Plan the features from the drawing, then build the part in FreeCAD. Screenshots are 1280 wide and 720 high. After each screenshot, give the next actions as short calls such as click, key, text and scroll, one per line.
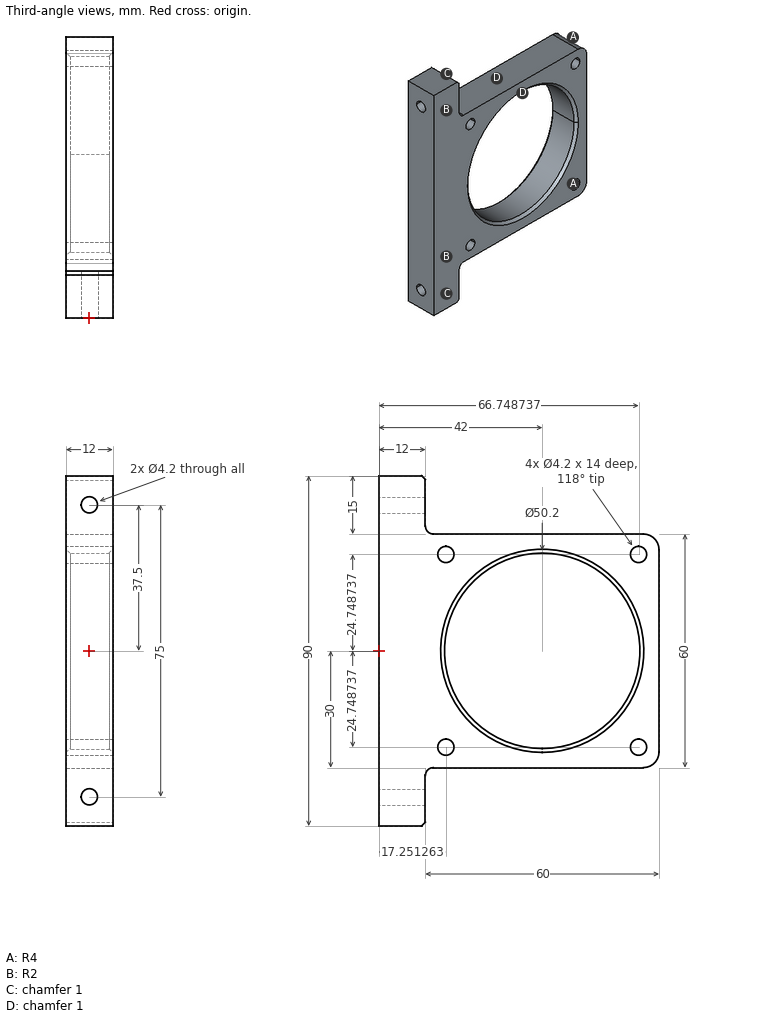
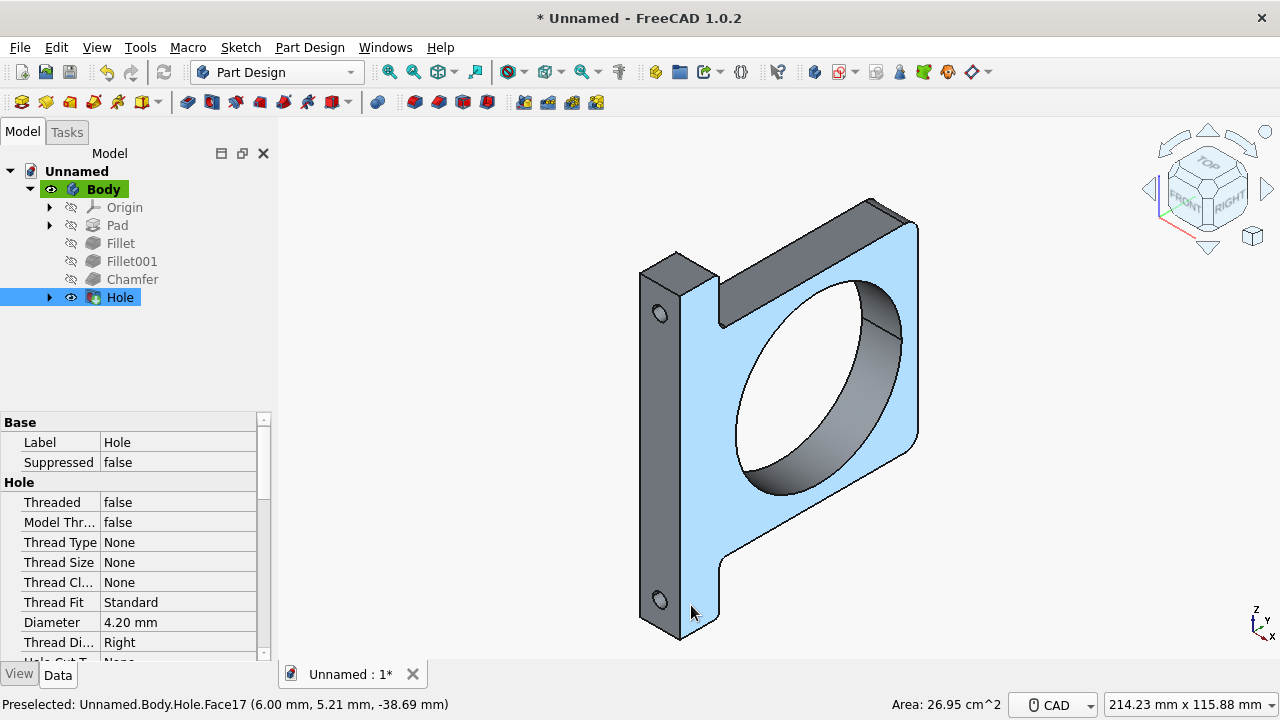
click(840, 72)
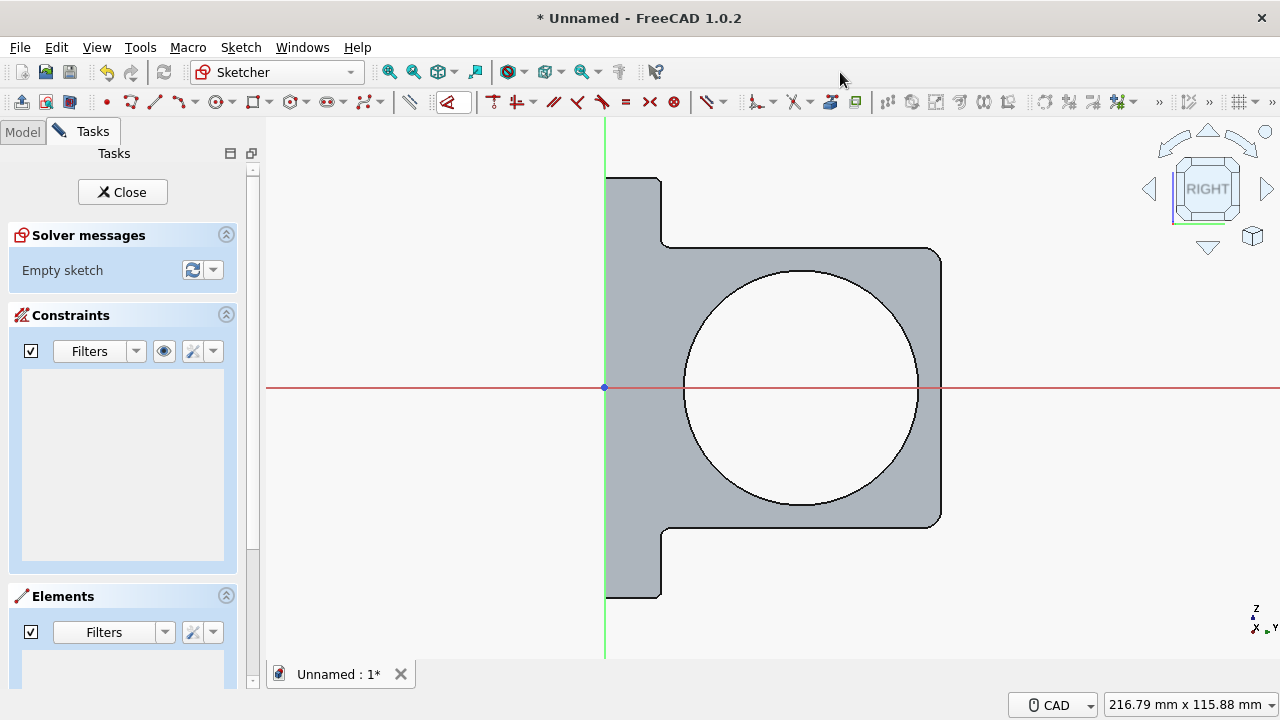
scroll(890, 388, up, 2)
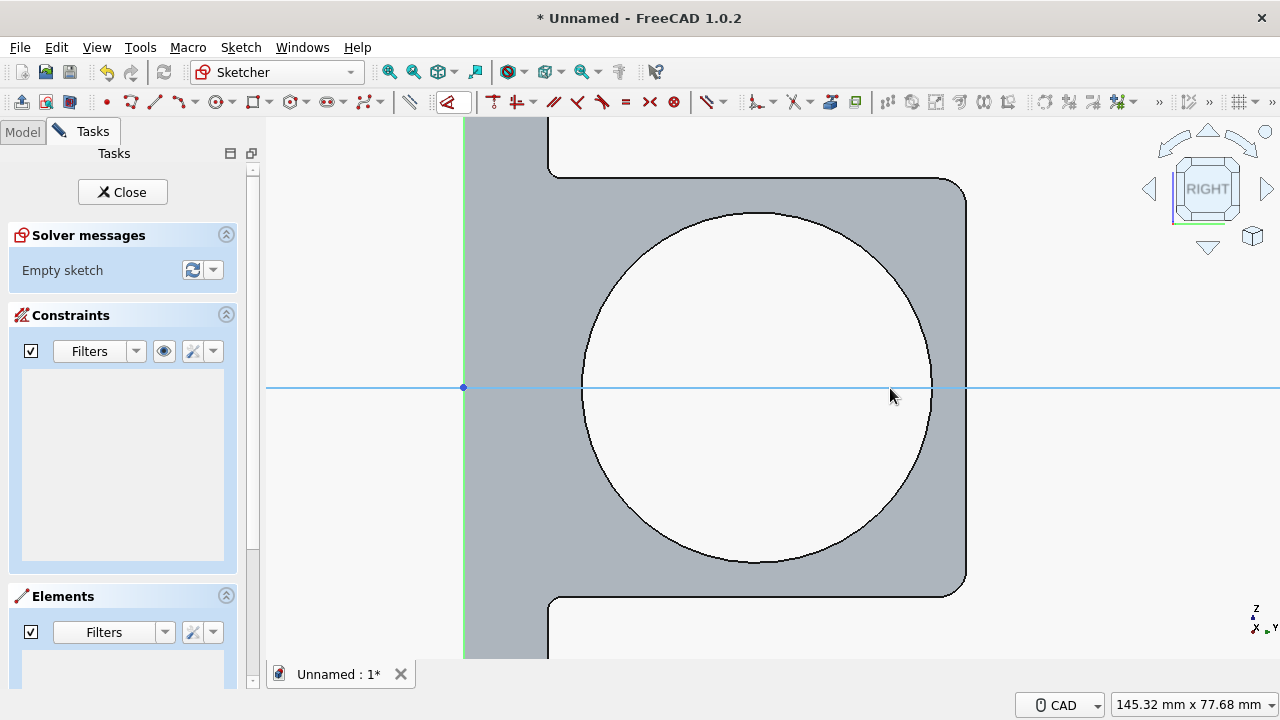
click(216, 102)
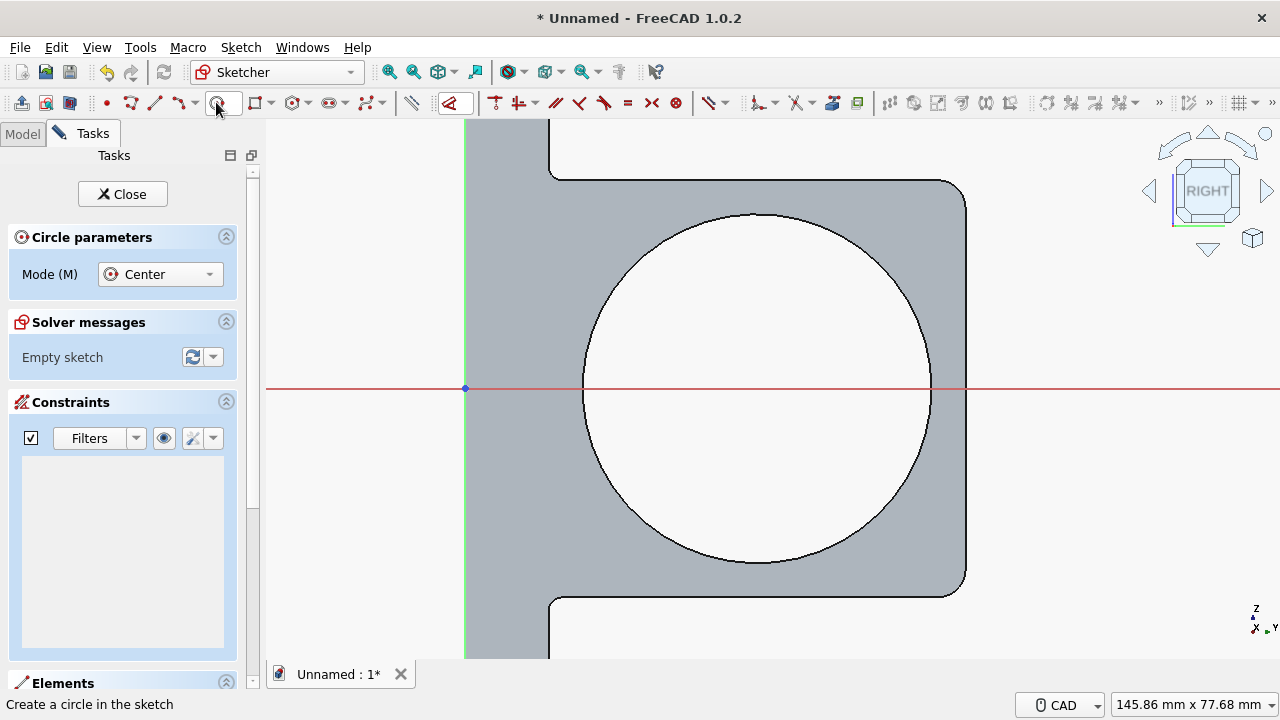
scroll(929, 217, up, 3)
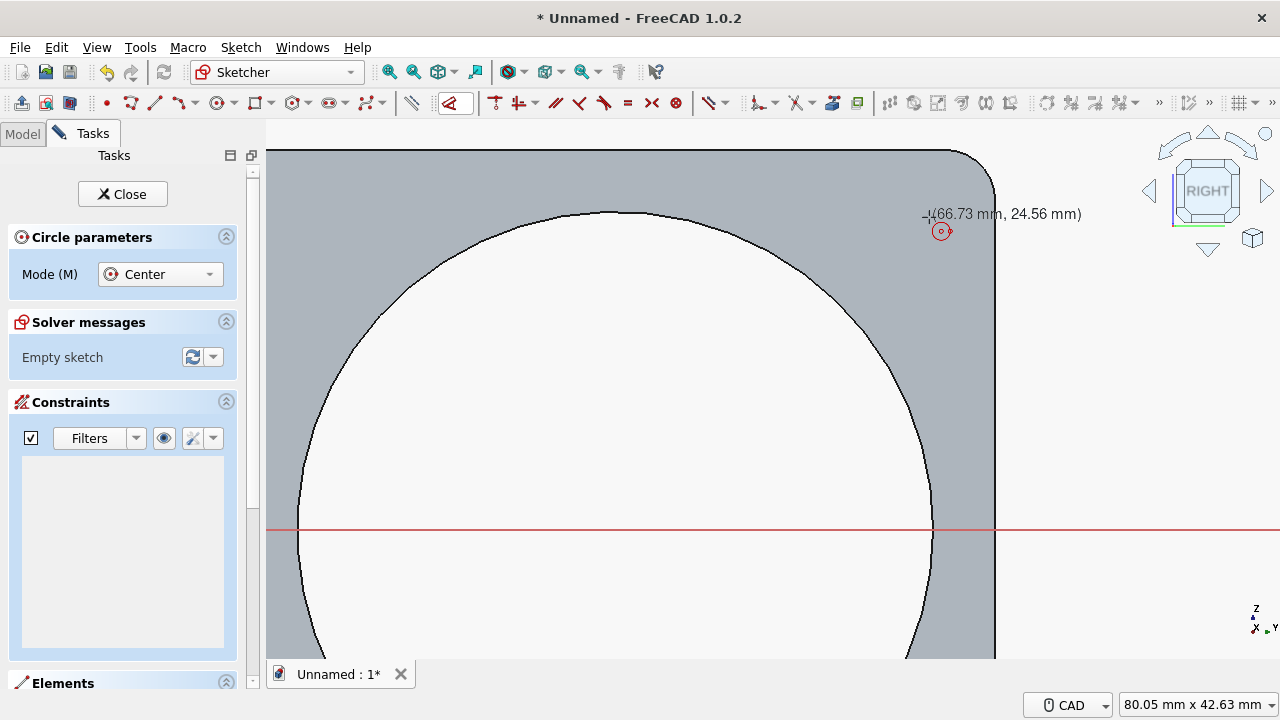
click(929, 216)
move(948, 197)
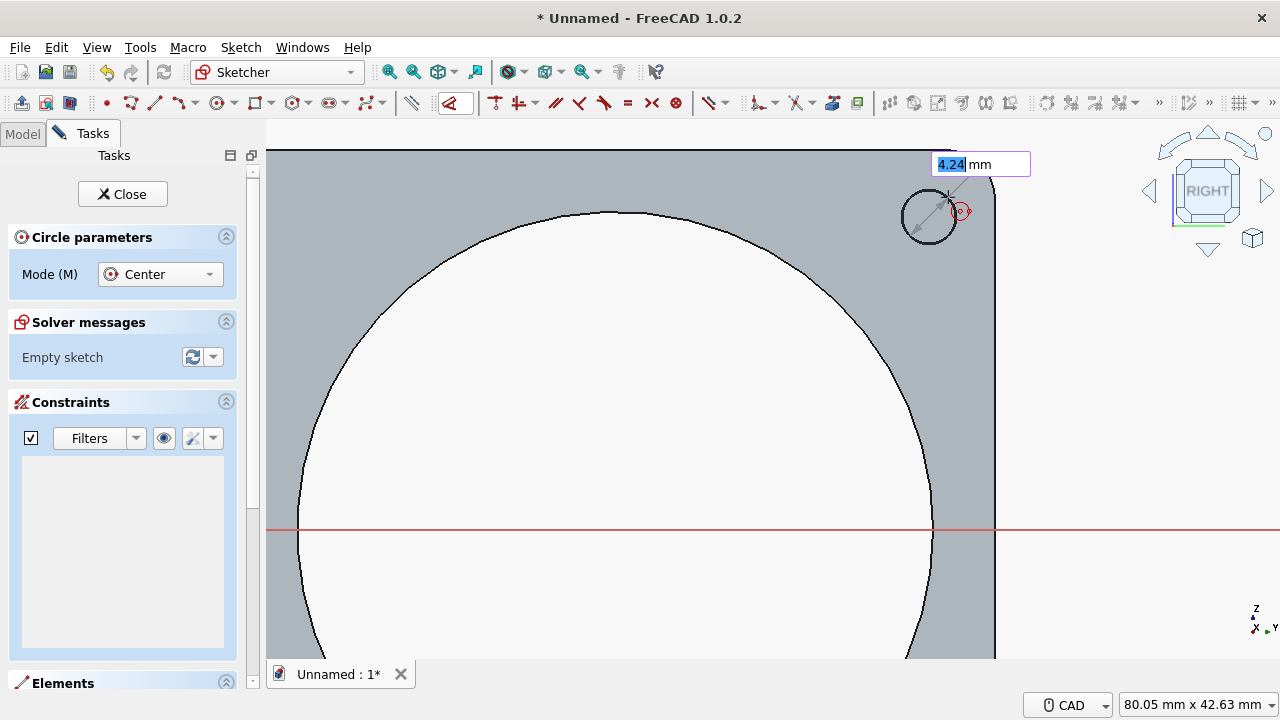
text(4.2)
key(Return)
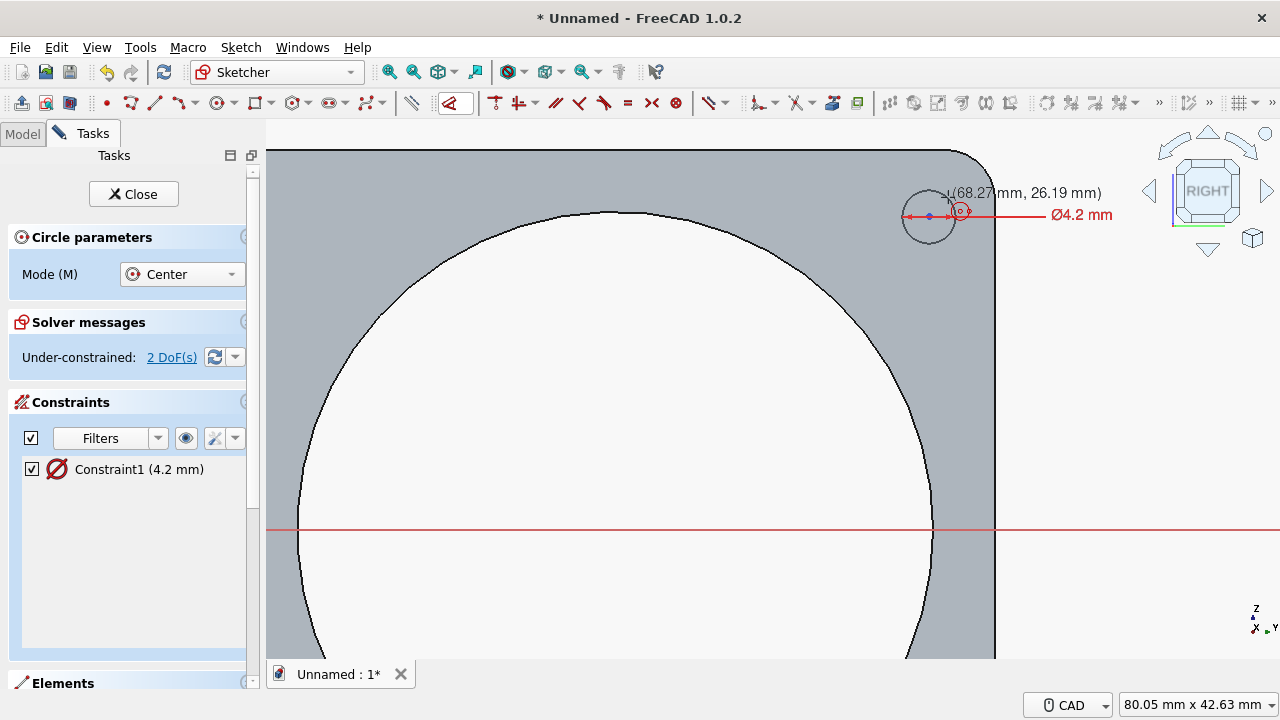
scroll(930, 218, down, 3)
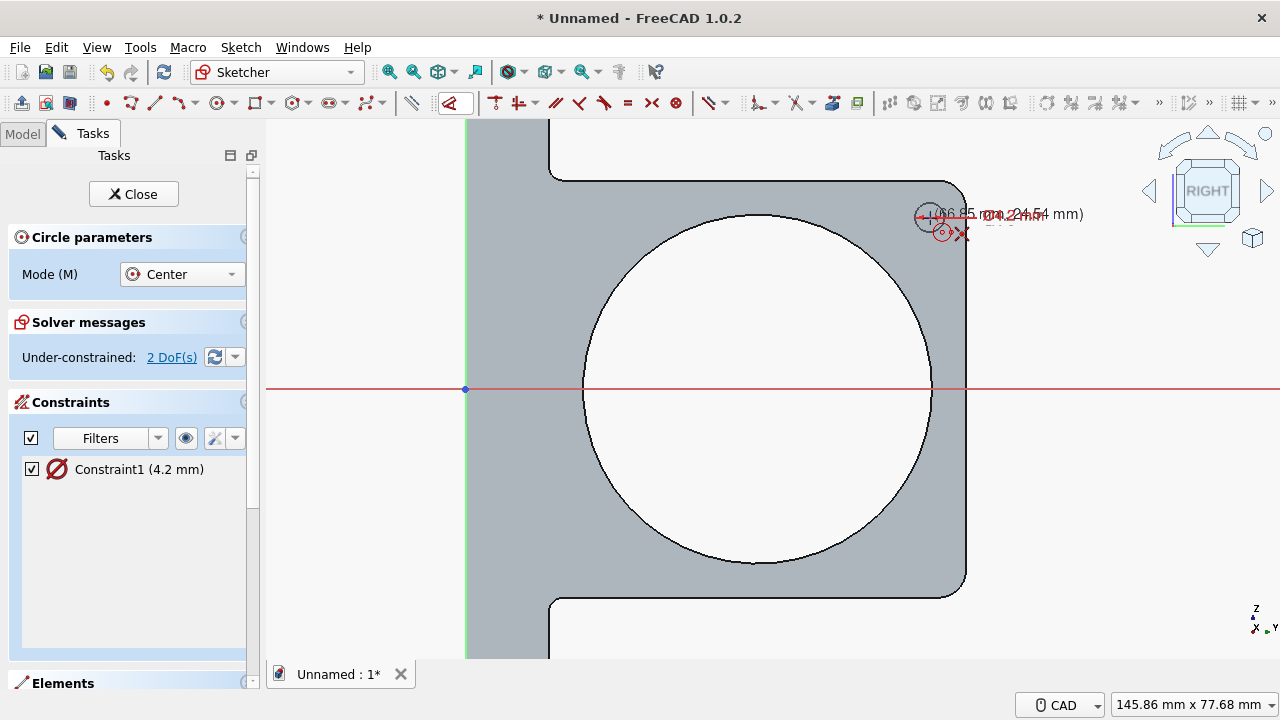
scroll(930, 561, up, 3)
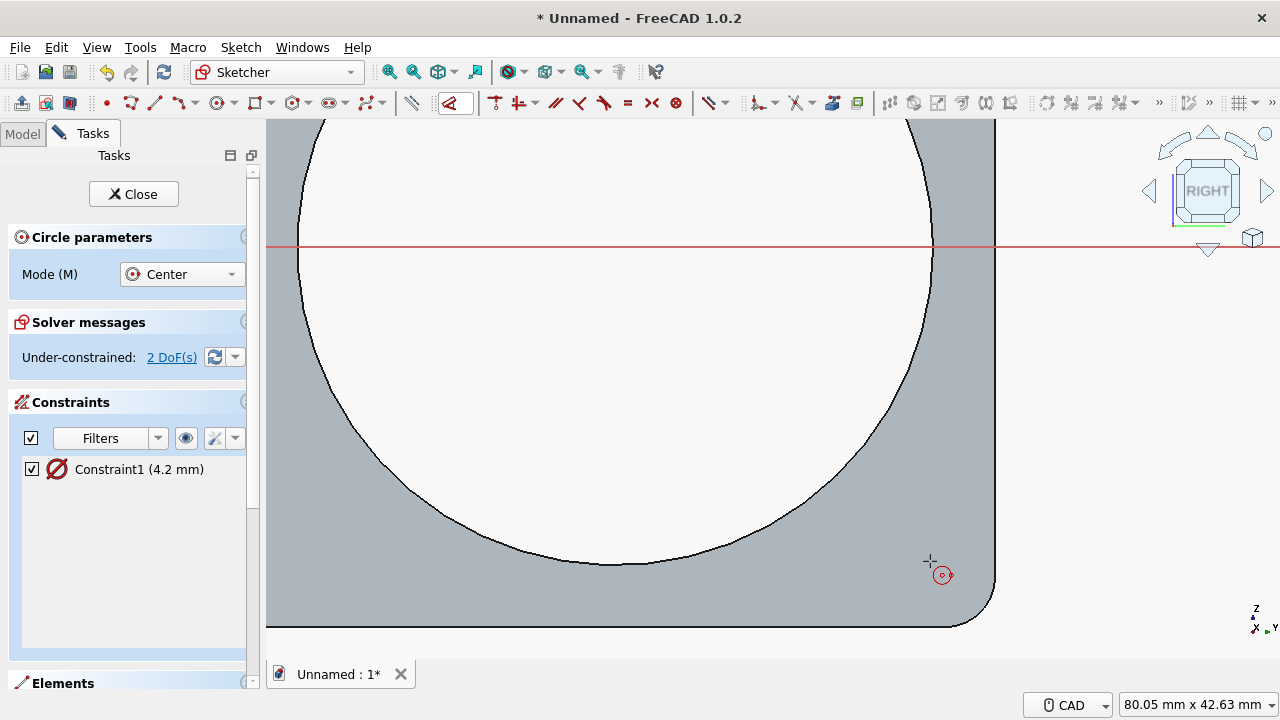
click(929, 561)
move(948, 542)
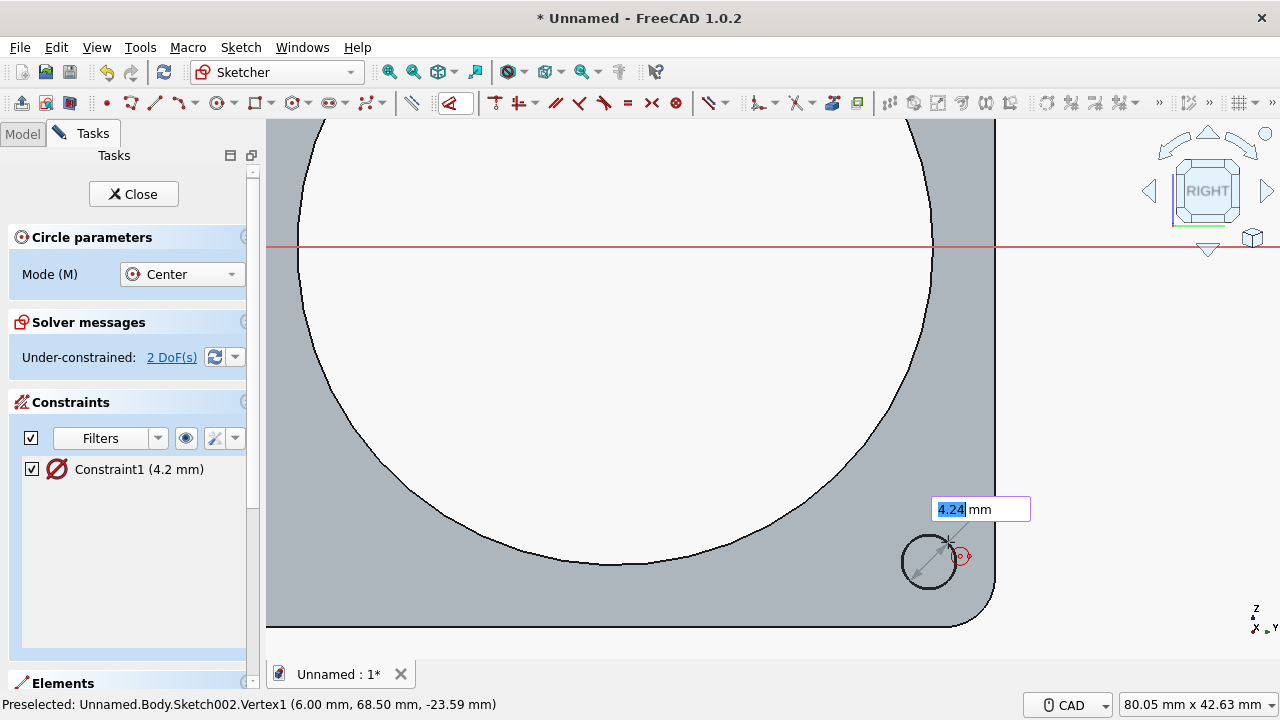
text(4.2)
key(Return)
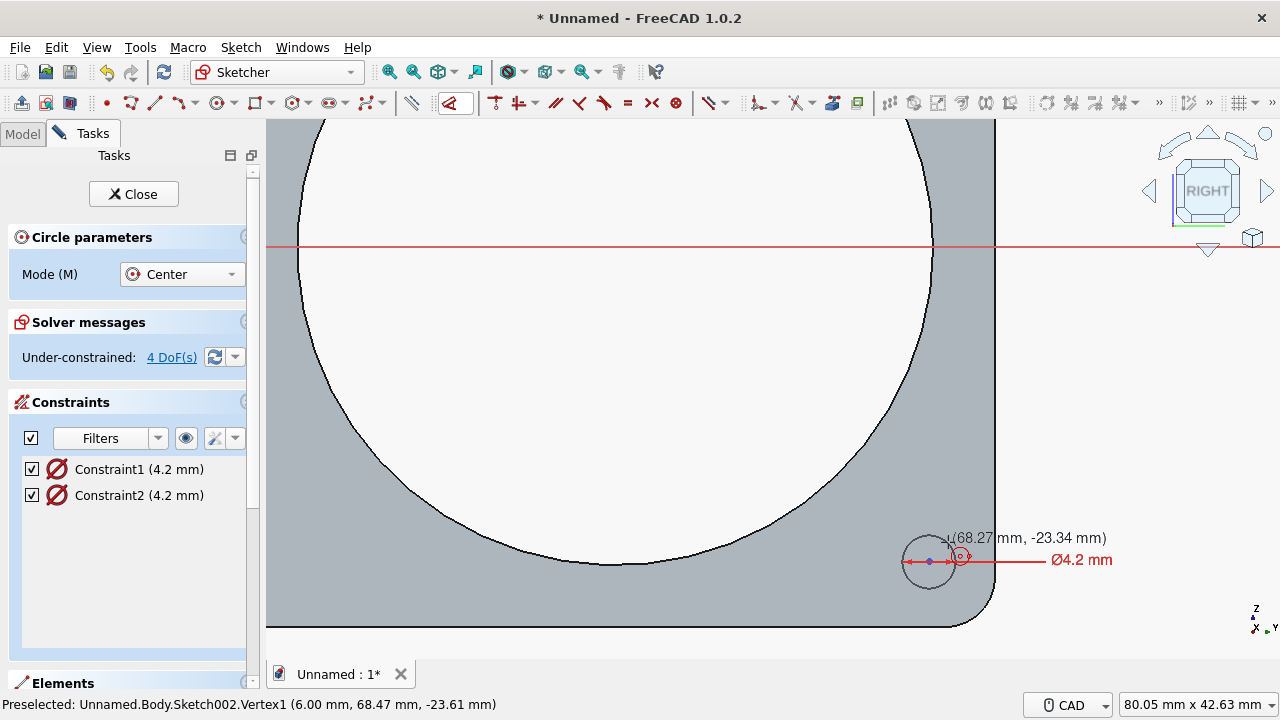
click(302, 561)
move(321, 542)